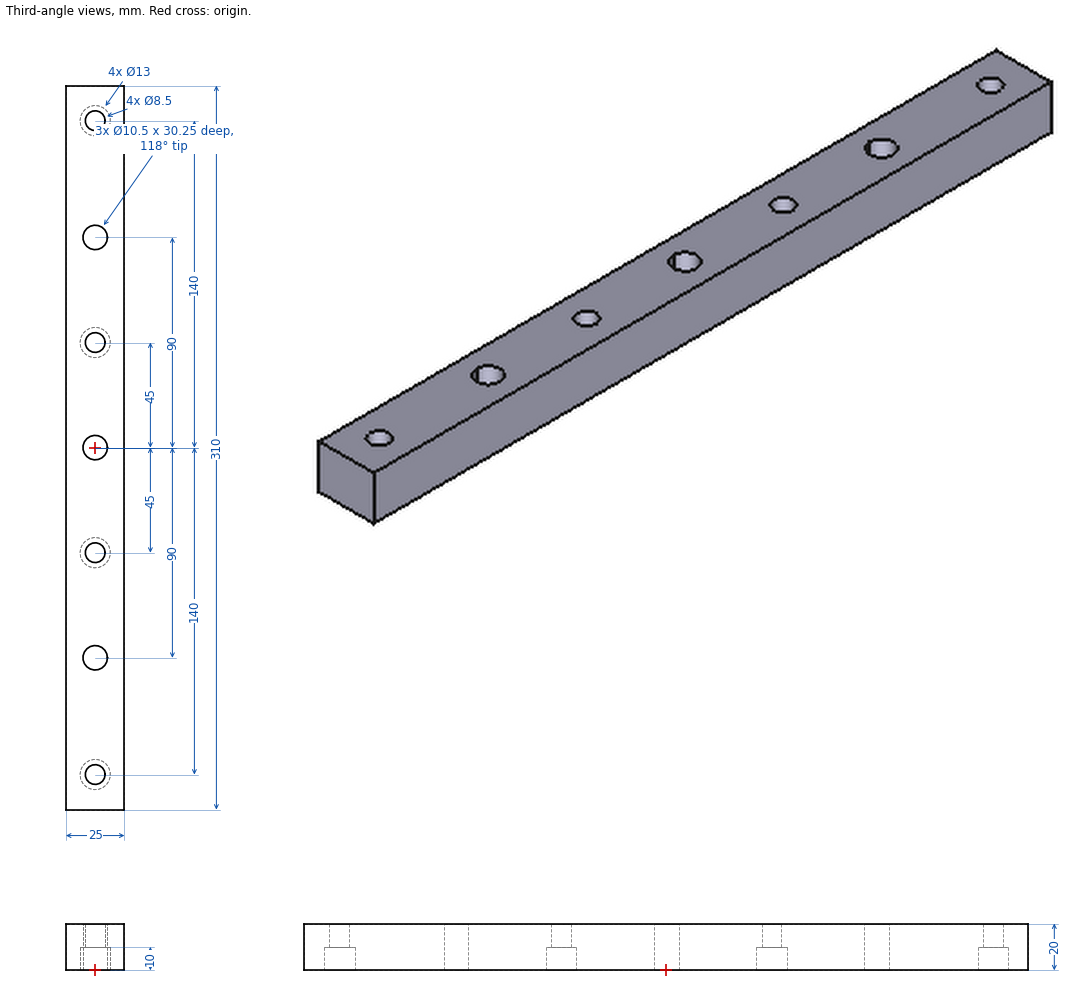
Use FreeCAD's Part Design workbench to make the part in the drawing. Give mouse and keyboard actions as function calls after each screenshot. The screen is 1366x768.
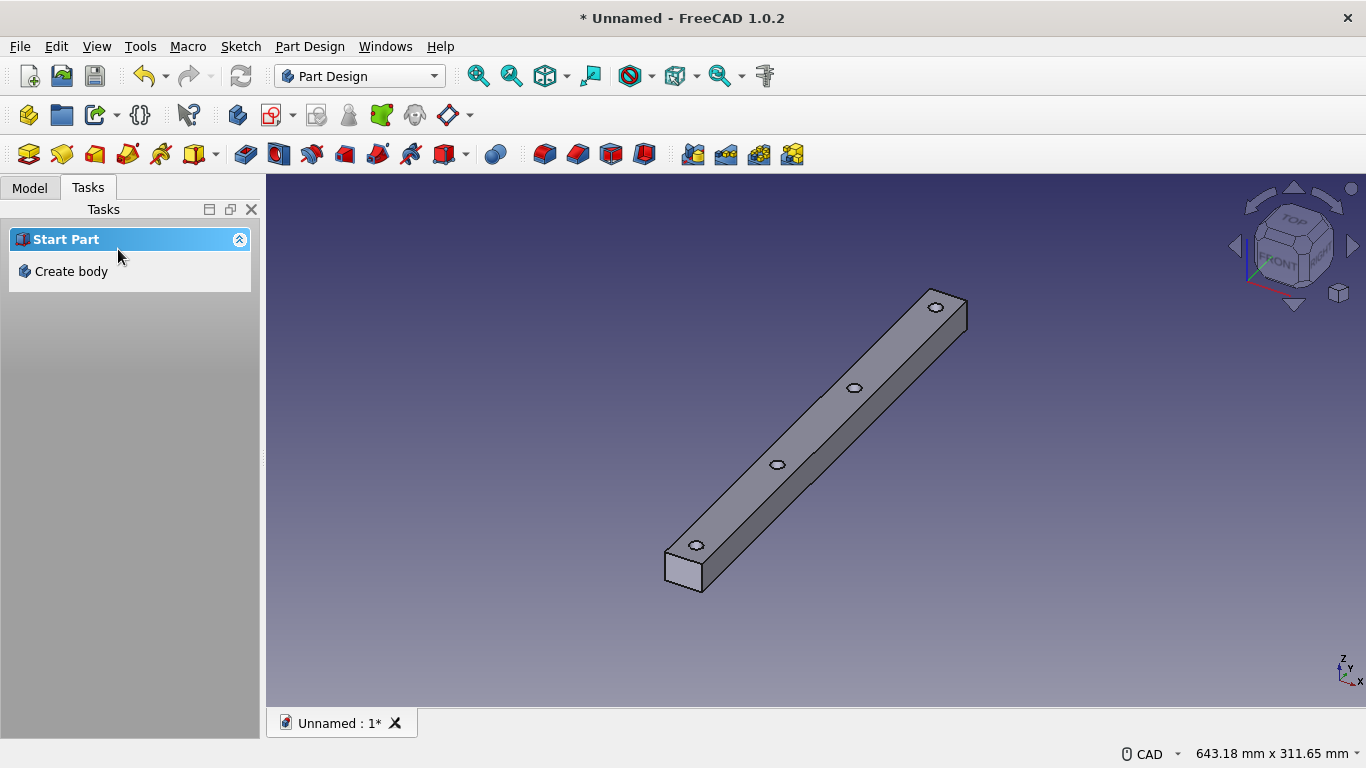
click(270, 116)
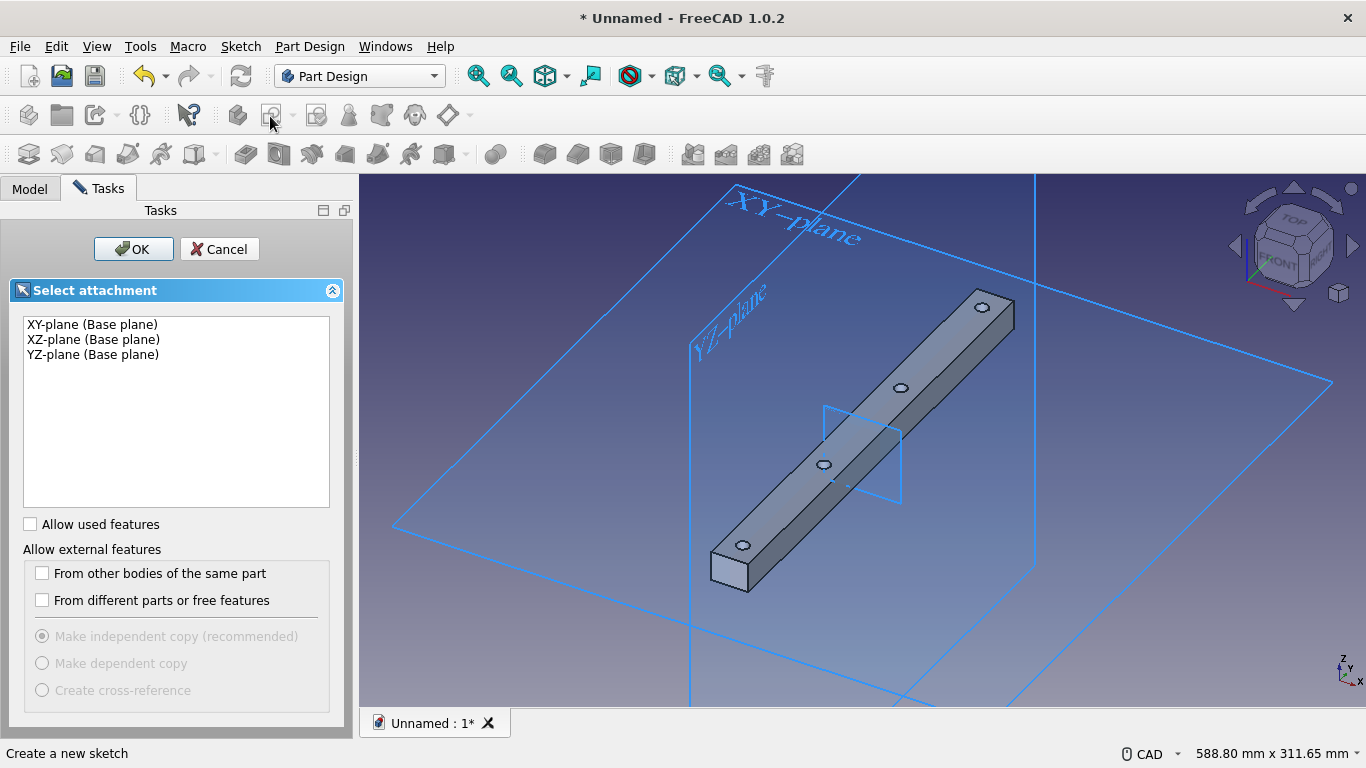
click(84, 324)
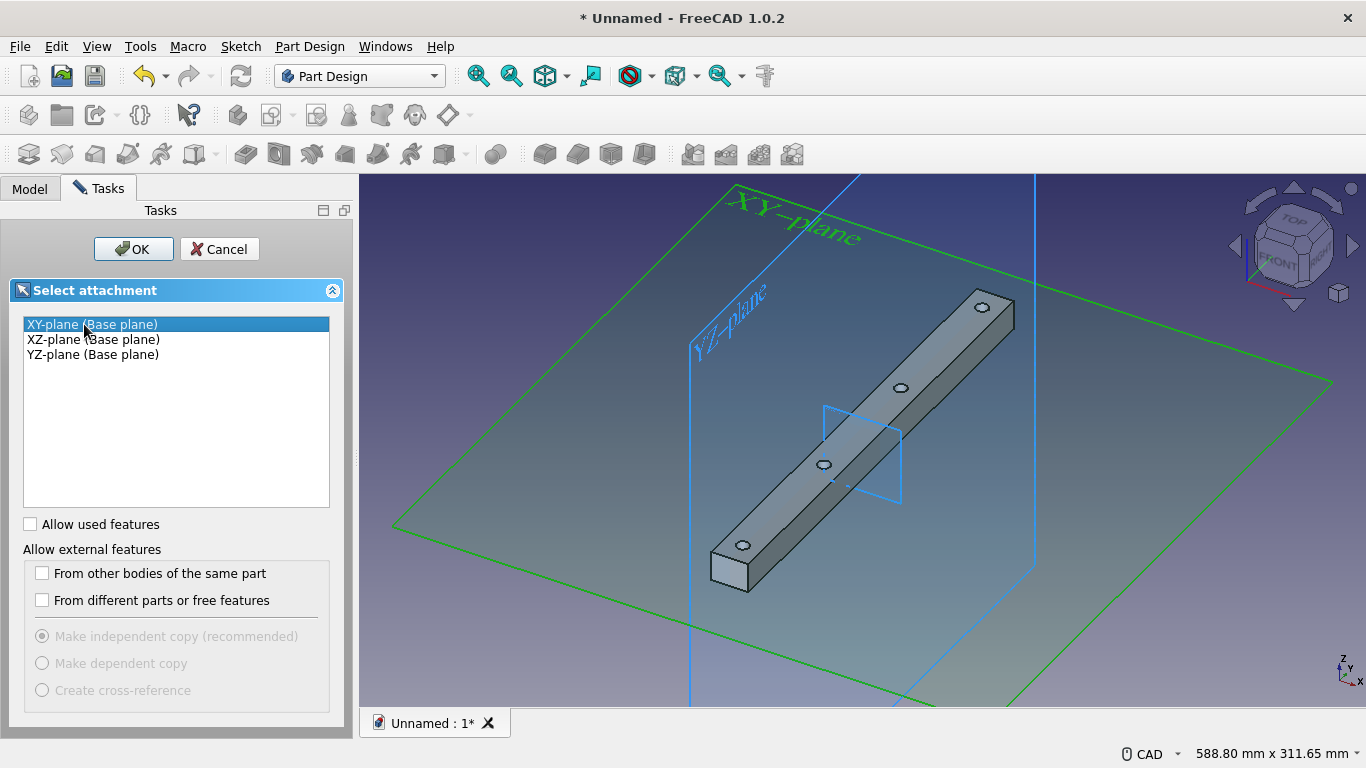
click(134, 249)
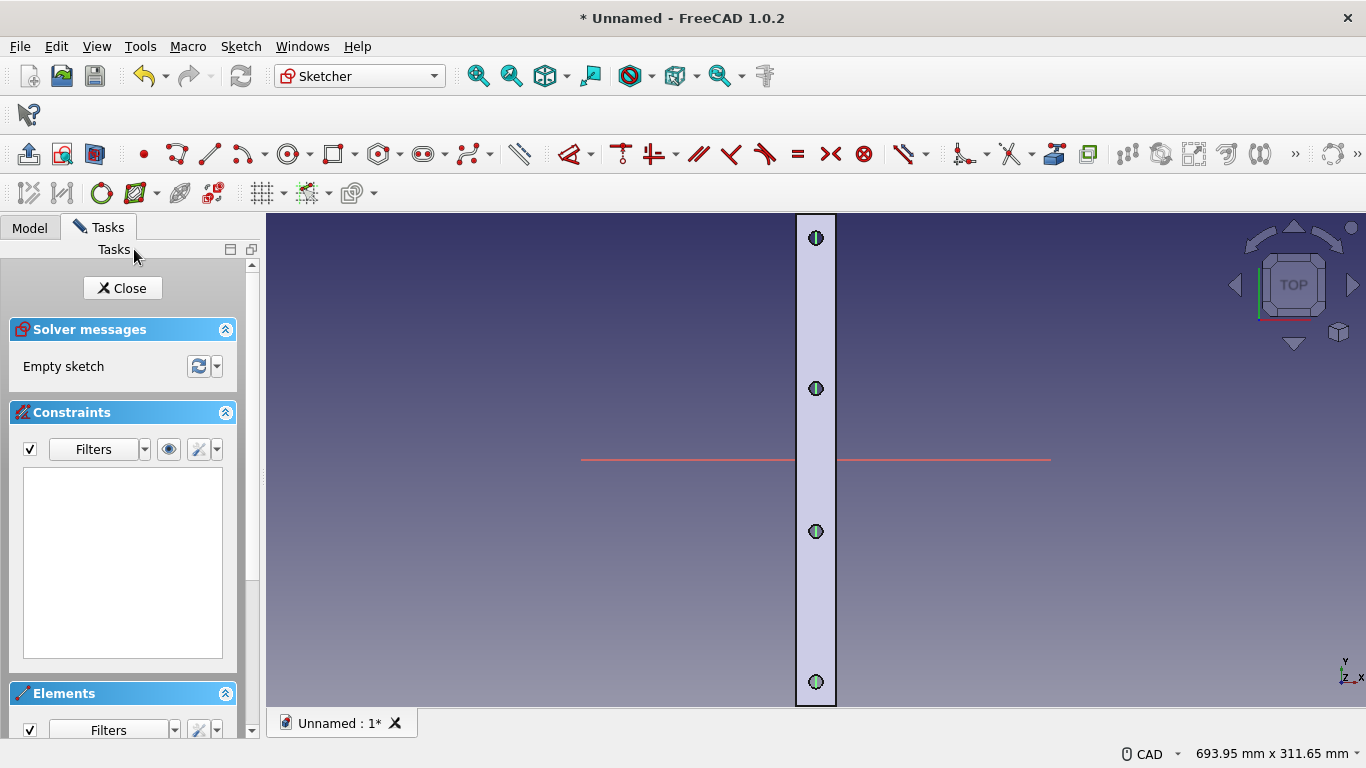
key(q)
key(s)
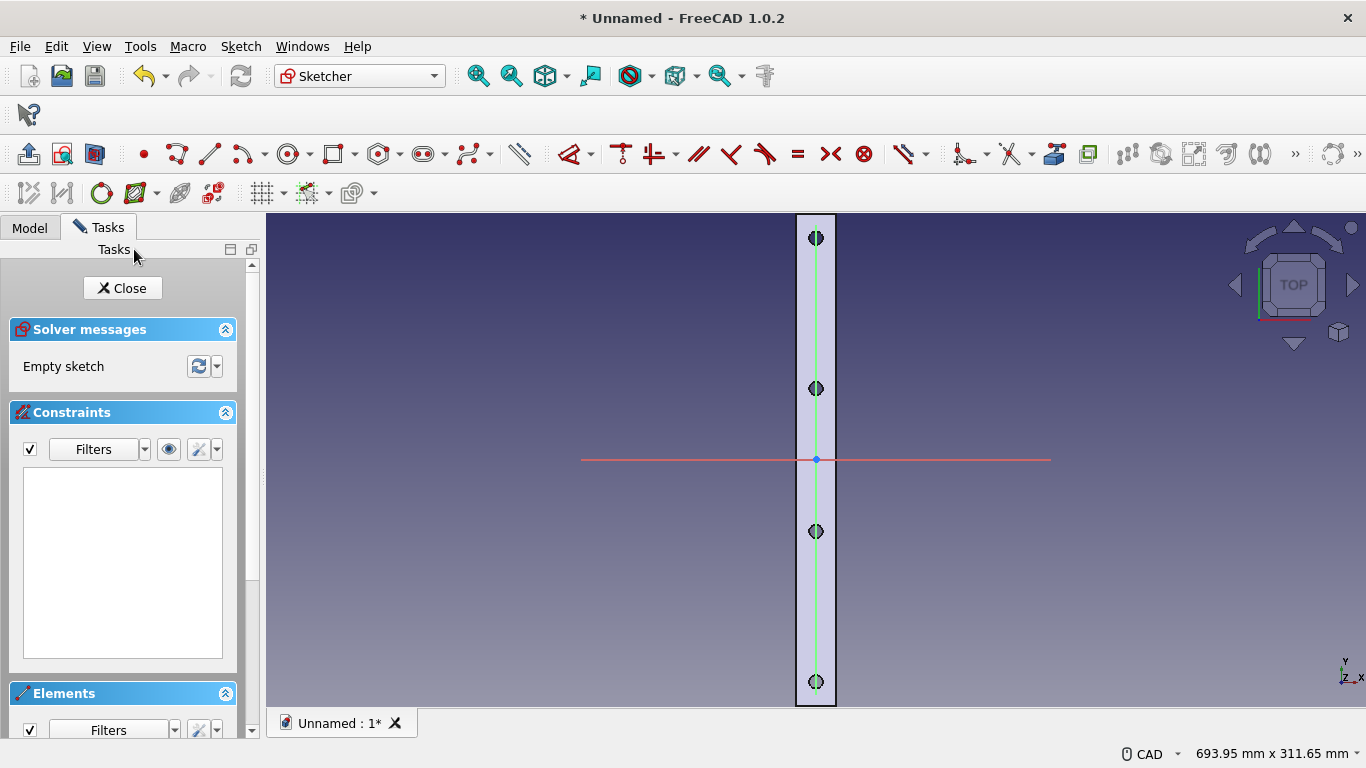
scroll(608, 460, down, 2)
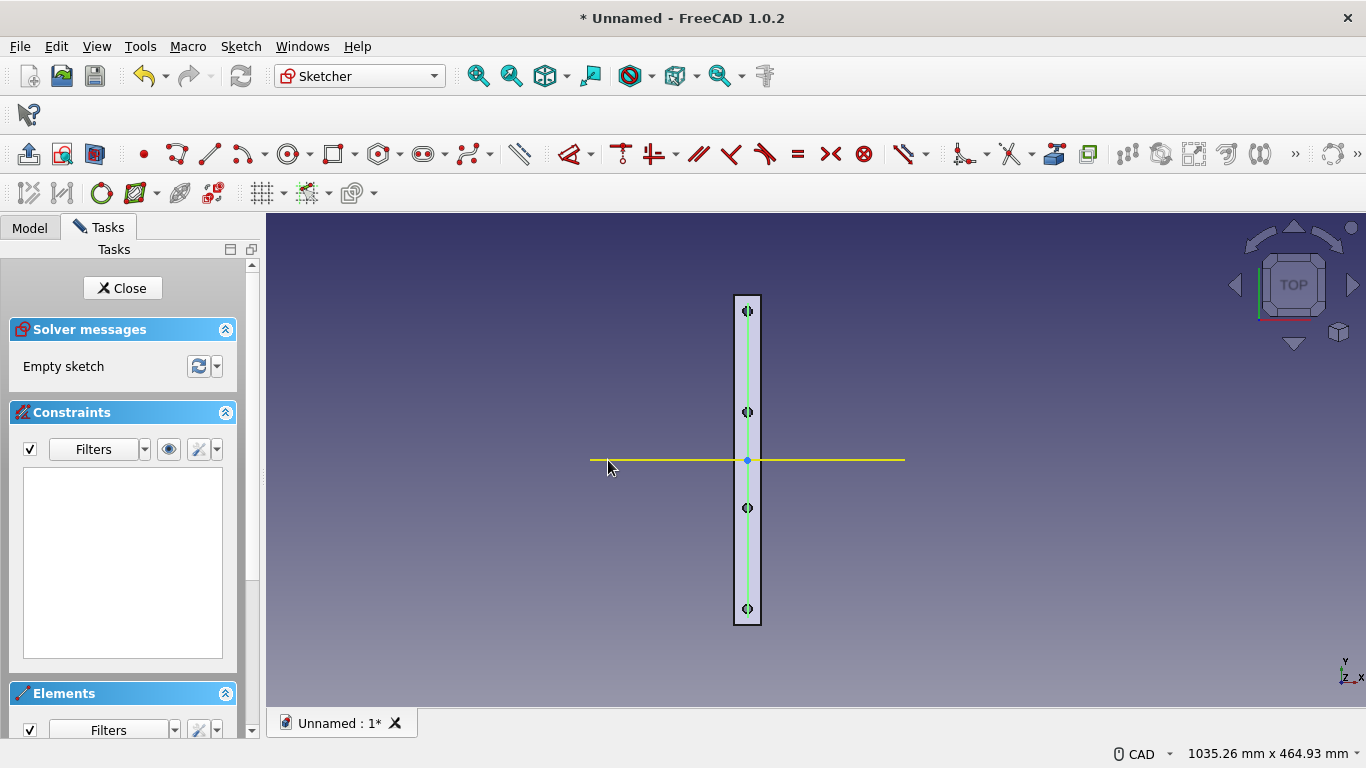
key(g)
key(c)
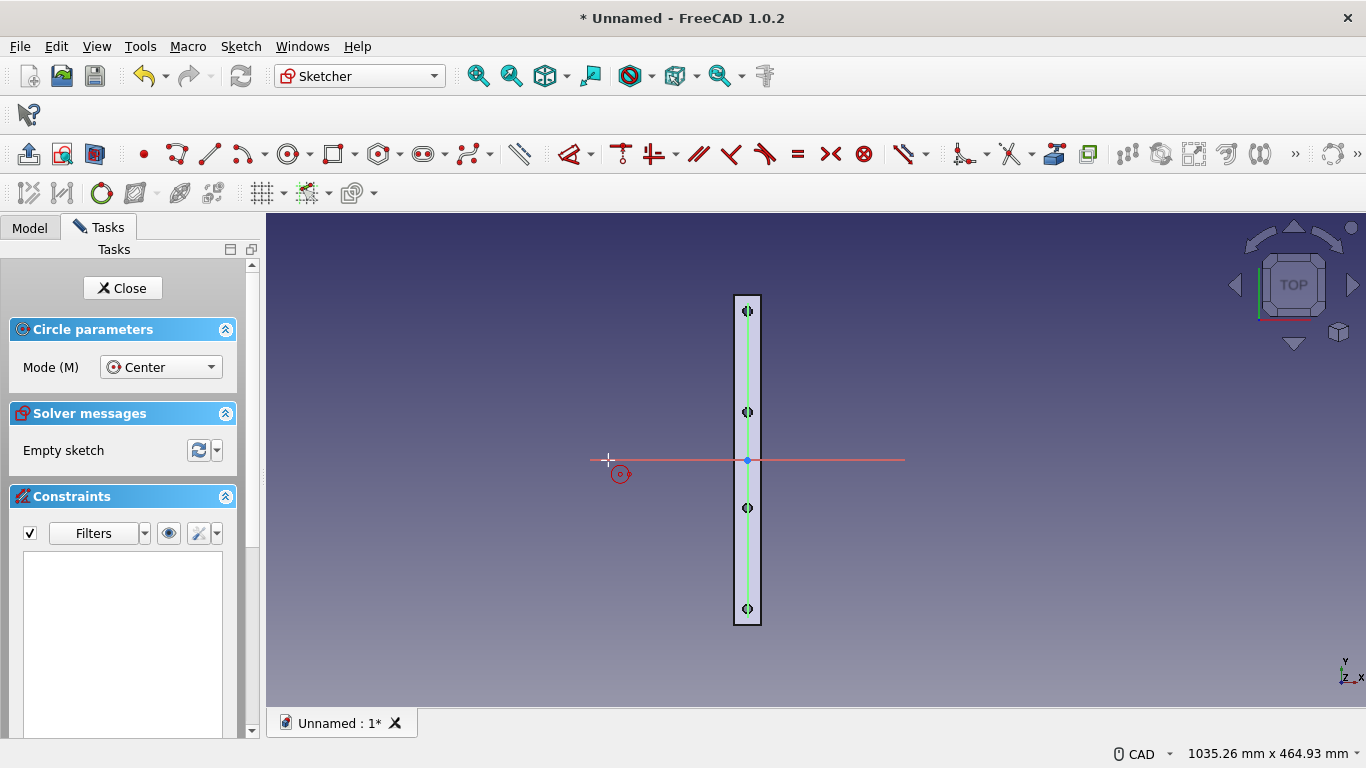
scroll(748, 311, up, 6)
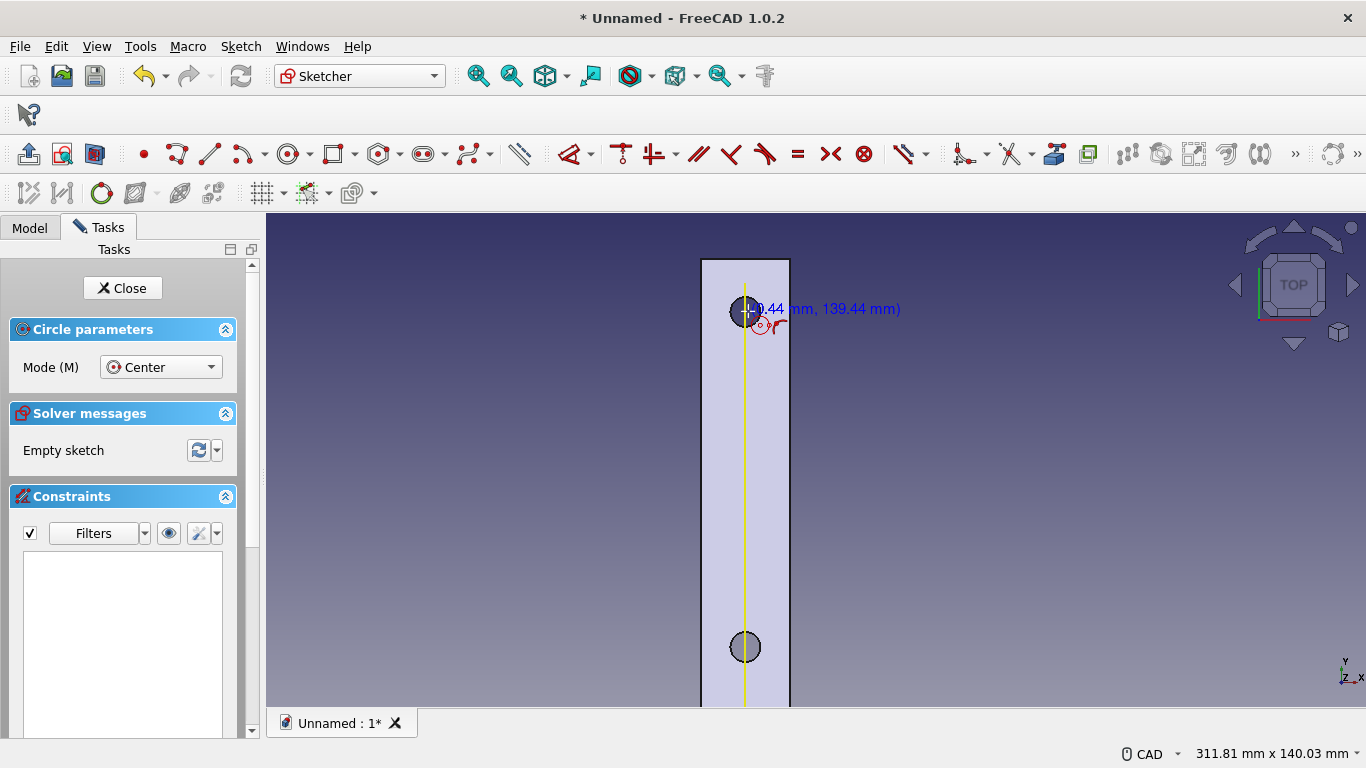
click(745, 312)
click(762, 296)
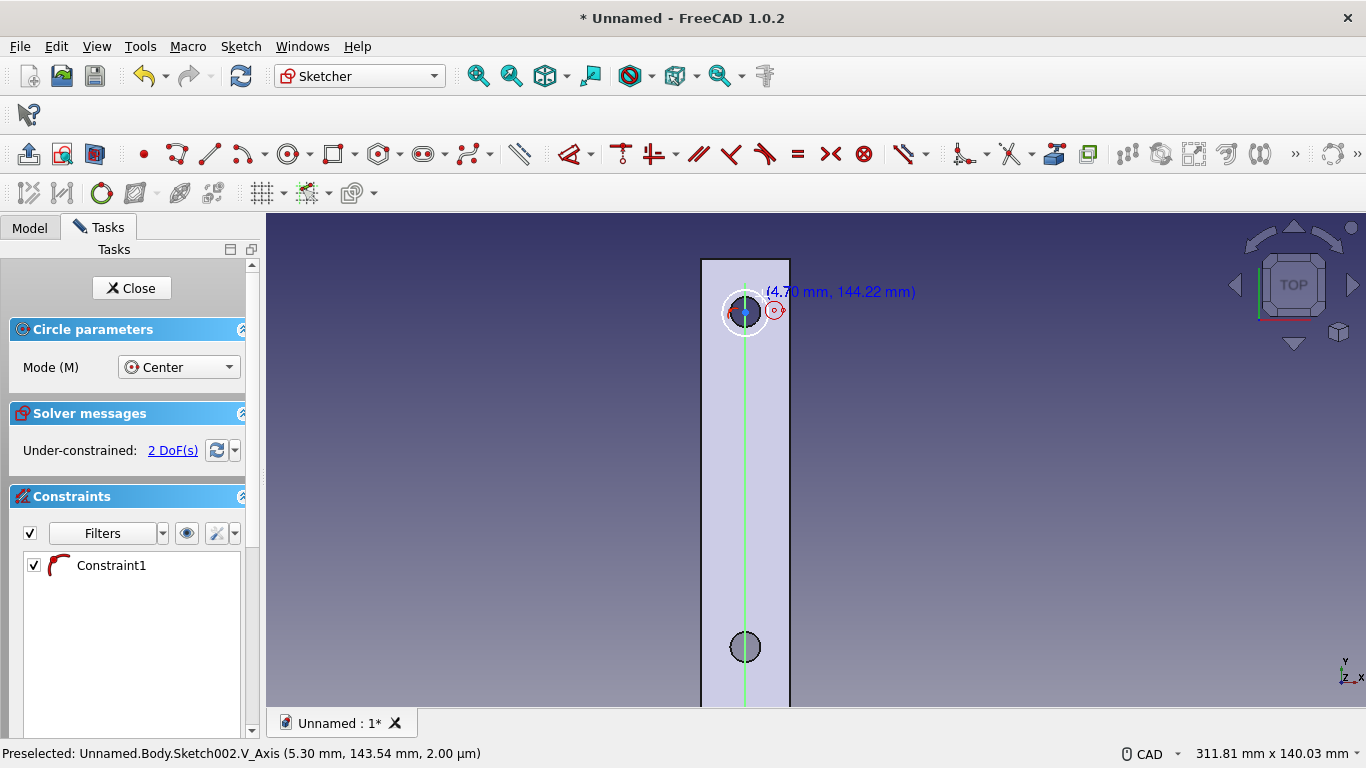
click(745, 647)
click(762, 631)